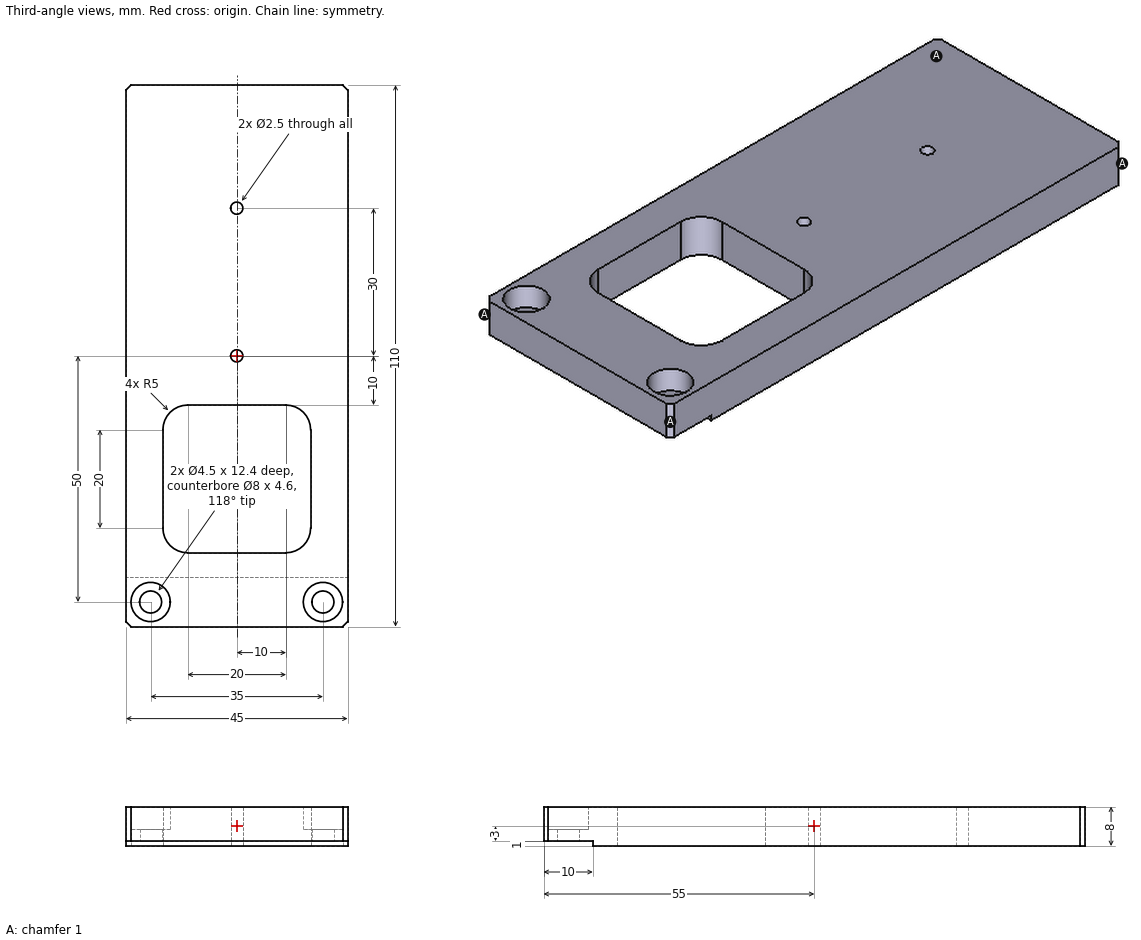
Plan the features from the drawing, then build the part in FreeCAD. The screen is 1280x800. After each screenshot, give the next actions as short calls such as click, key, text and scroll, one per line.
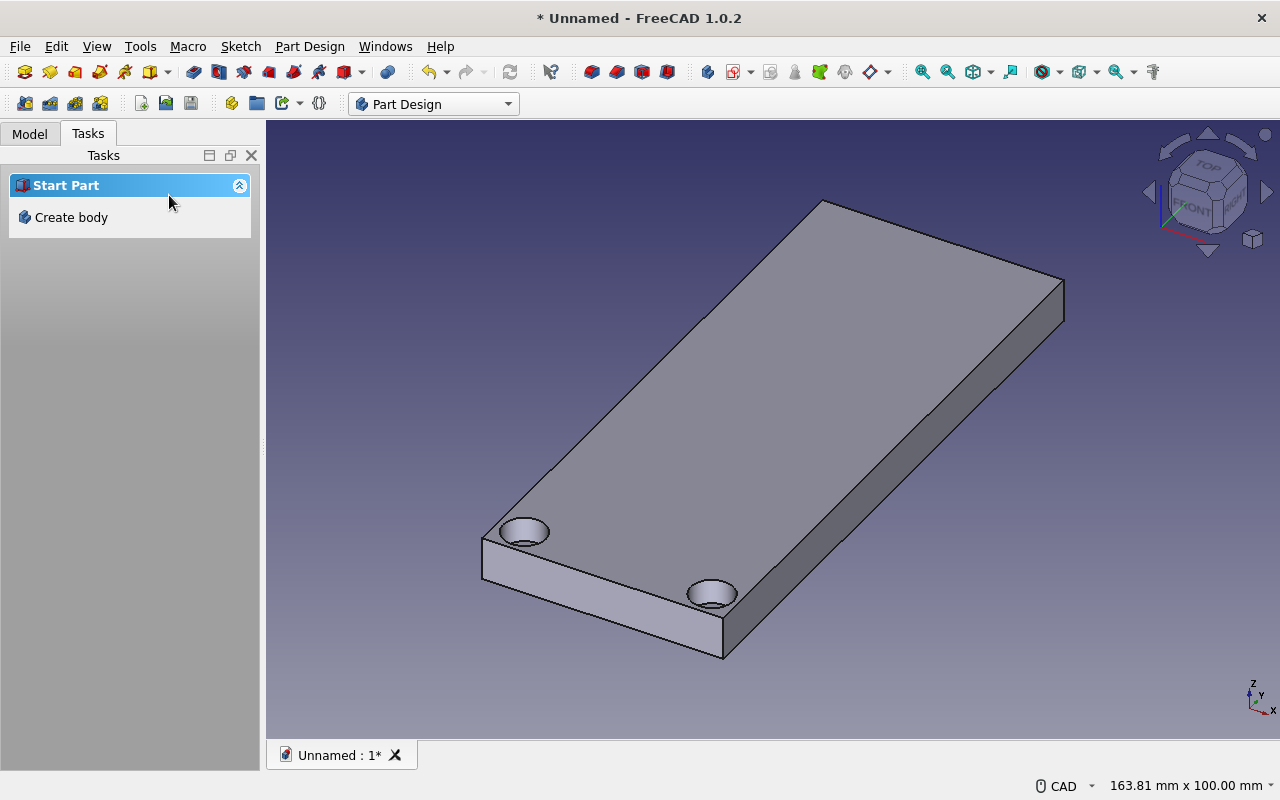
click(1040, 323)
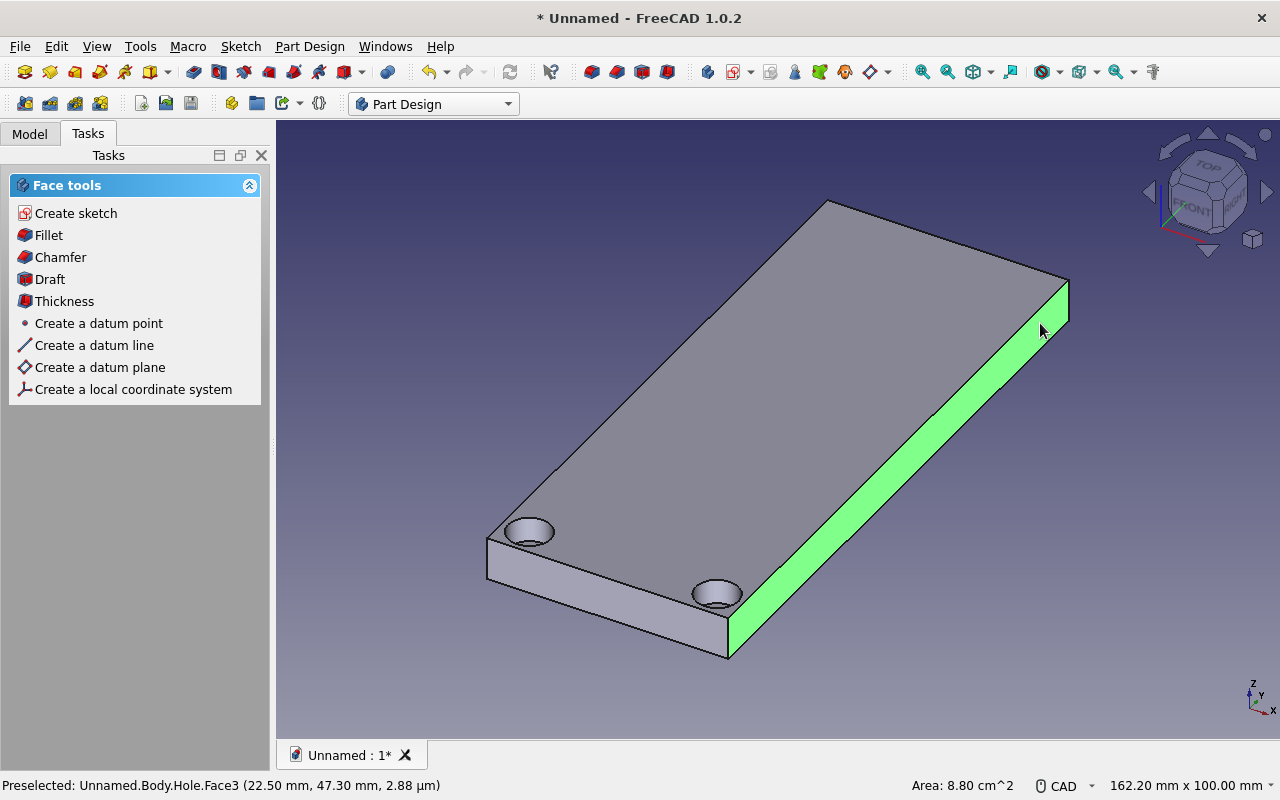
click(732, 72)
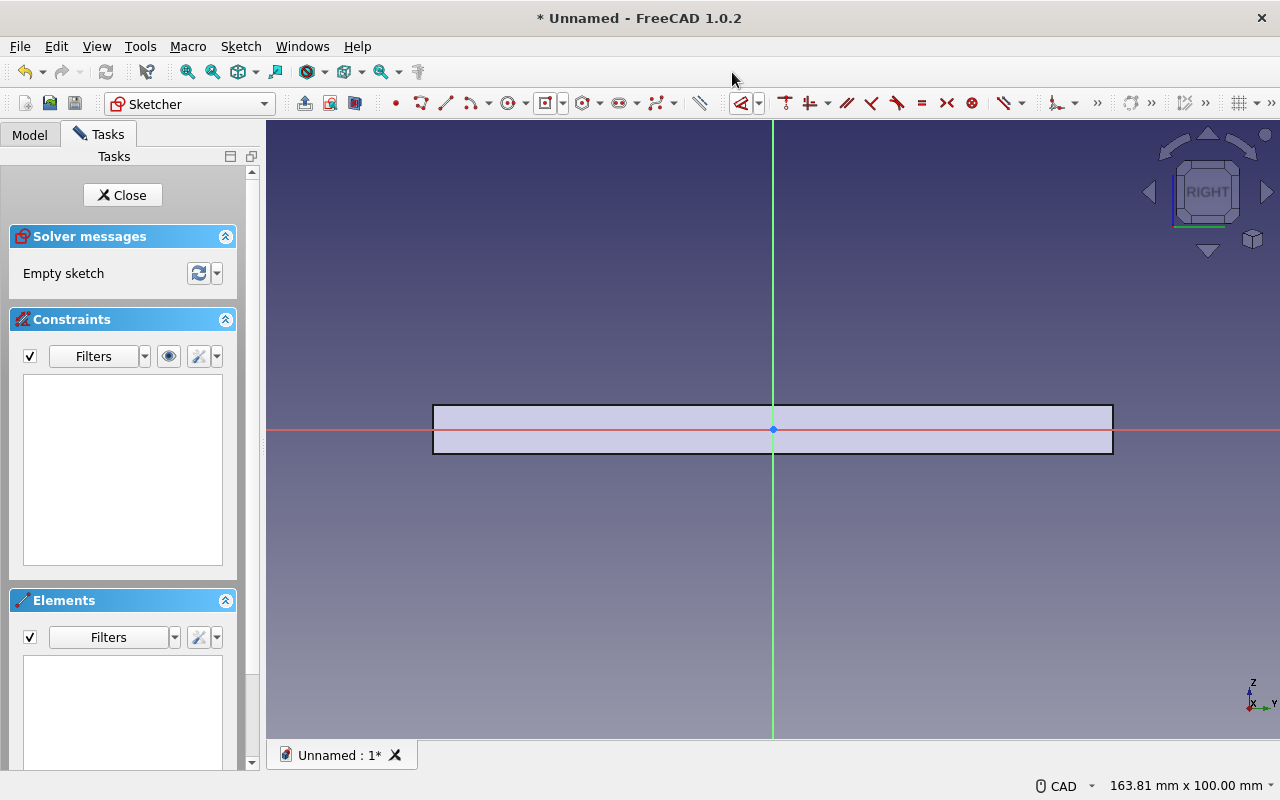
scroll(433, 454, up, 11)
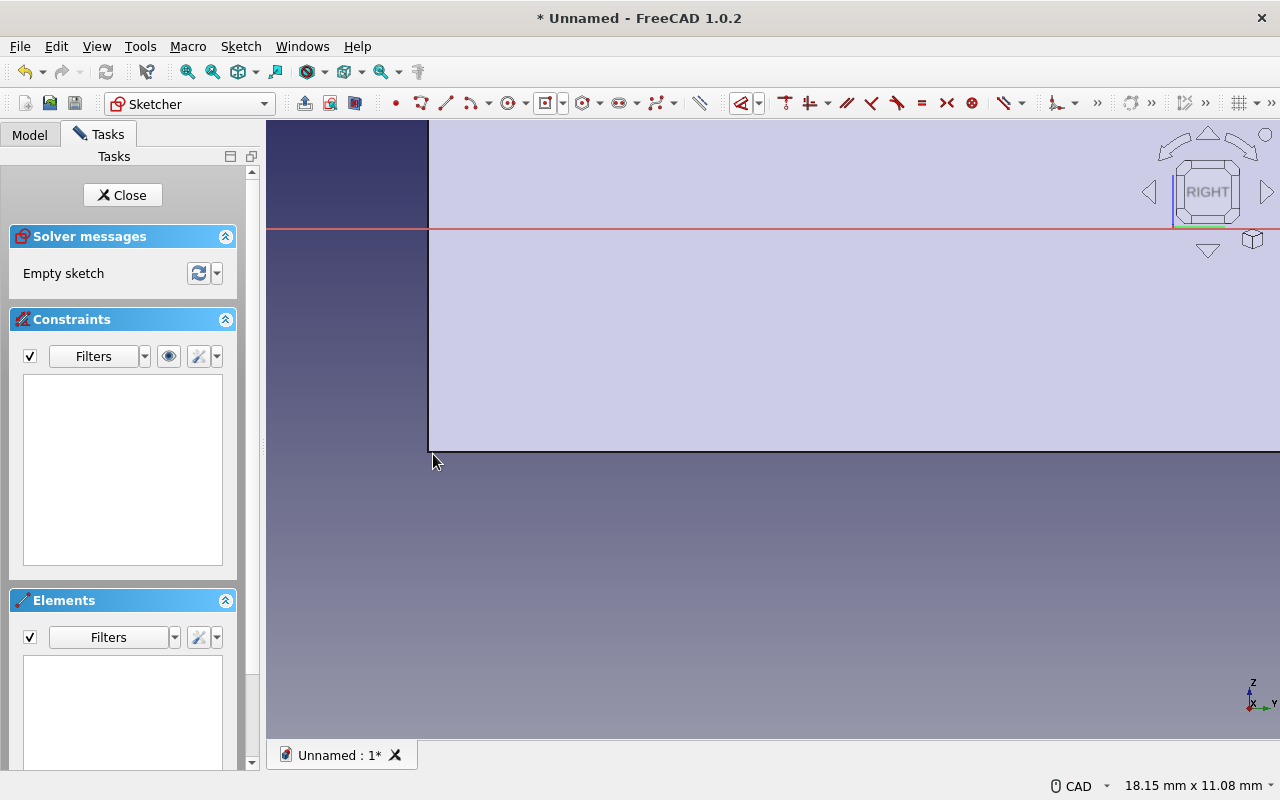
click(562, 104)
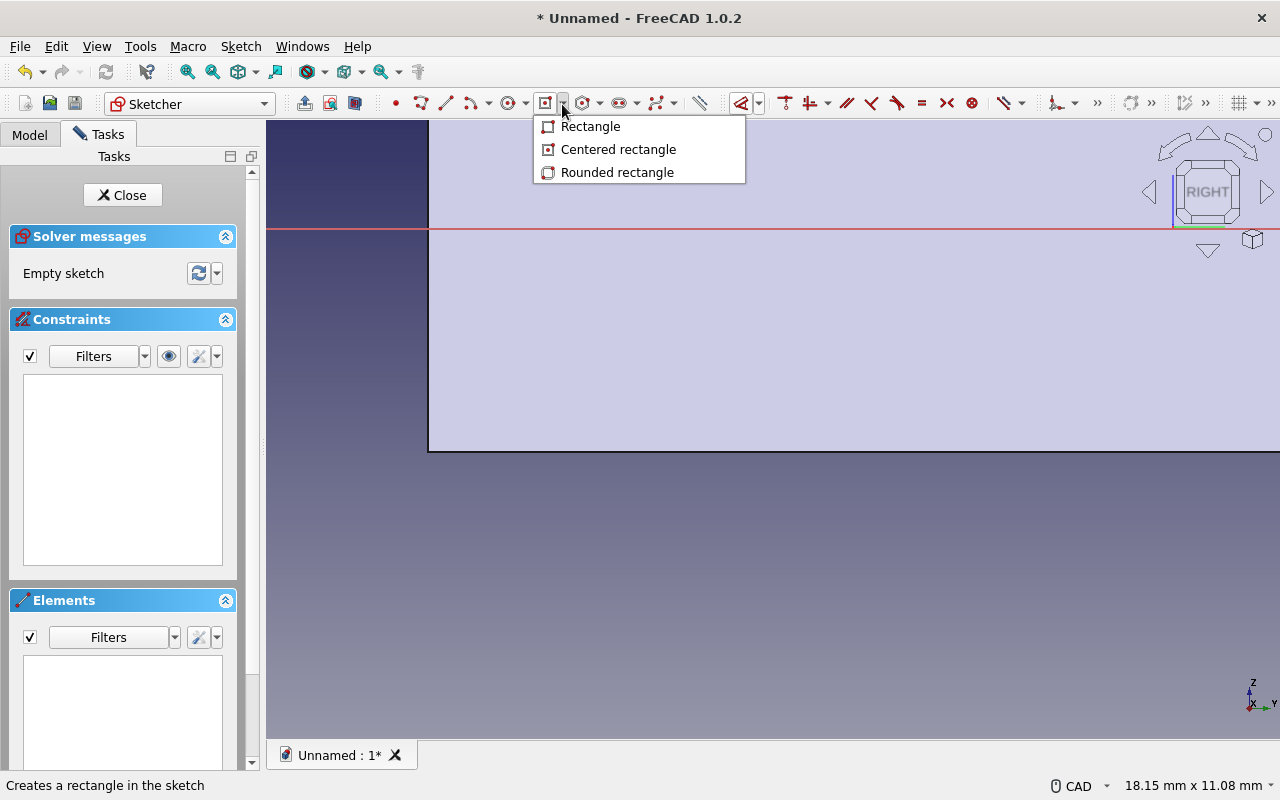
click(640, 126)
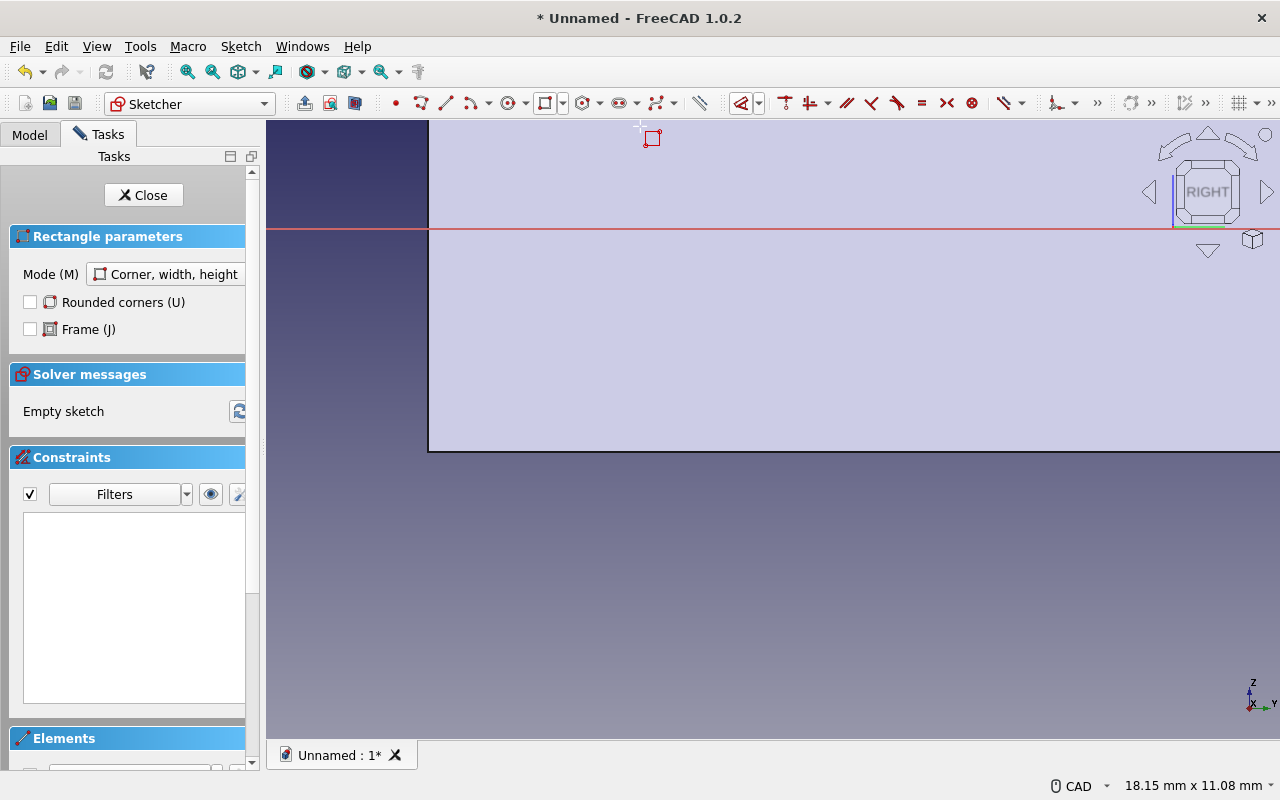
click(428, 396)
move(986, 452)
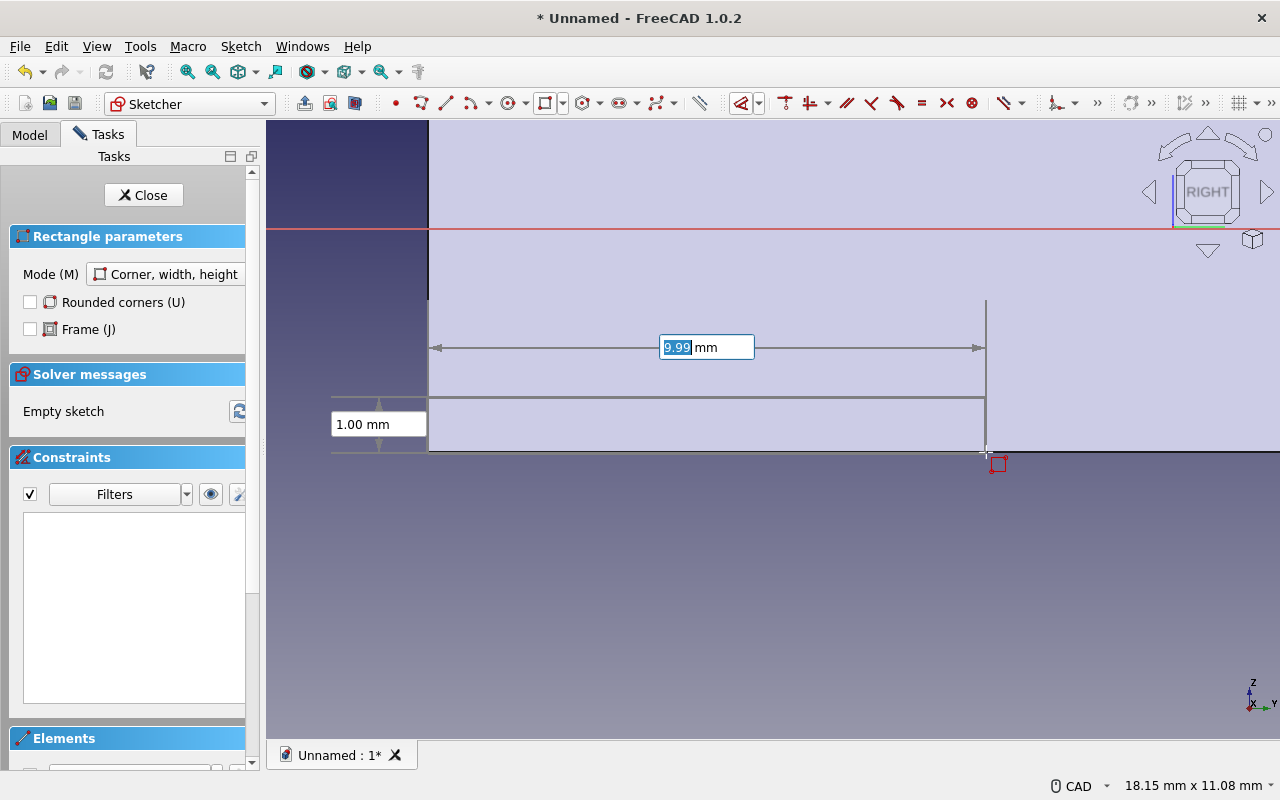
text(10)
key(Tab)
text(1)
key(Return)
key(Escape)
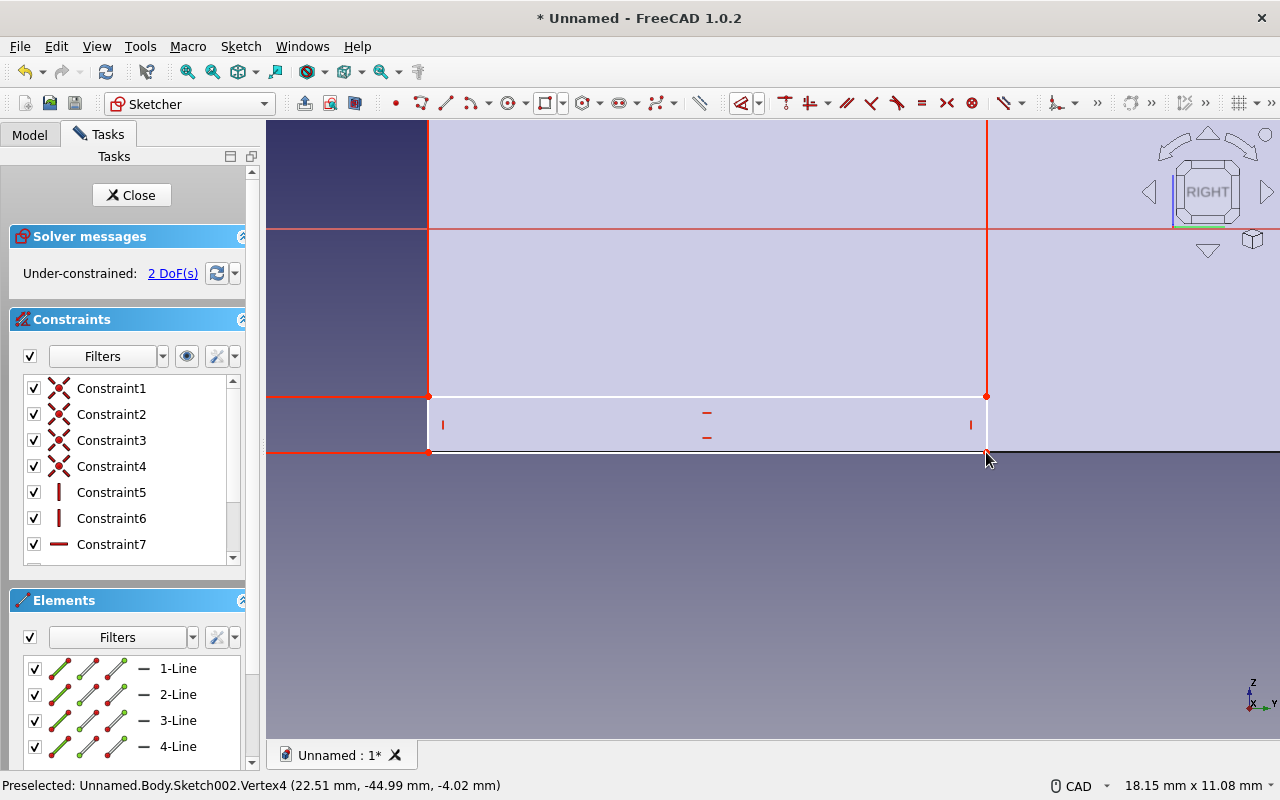
click(428, 397)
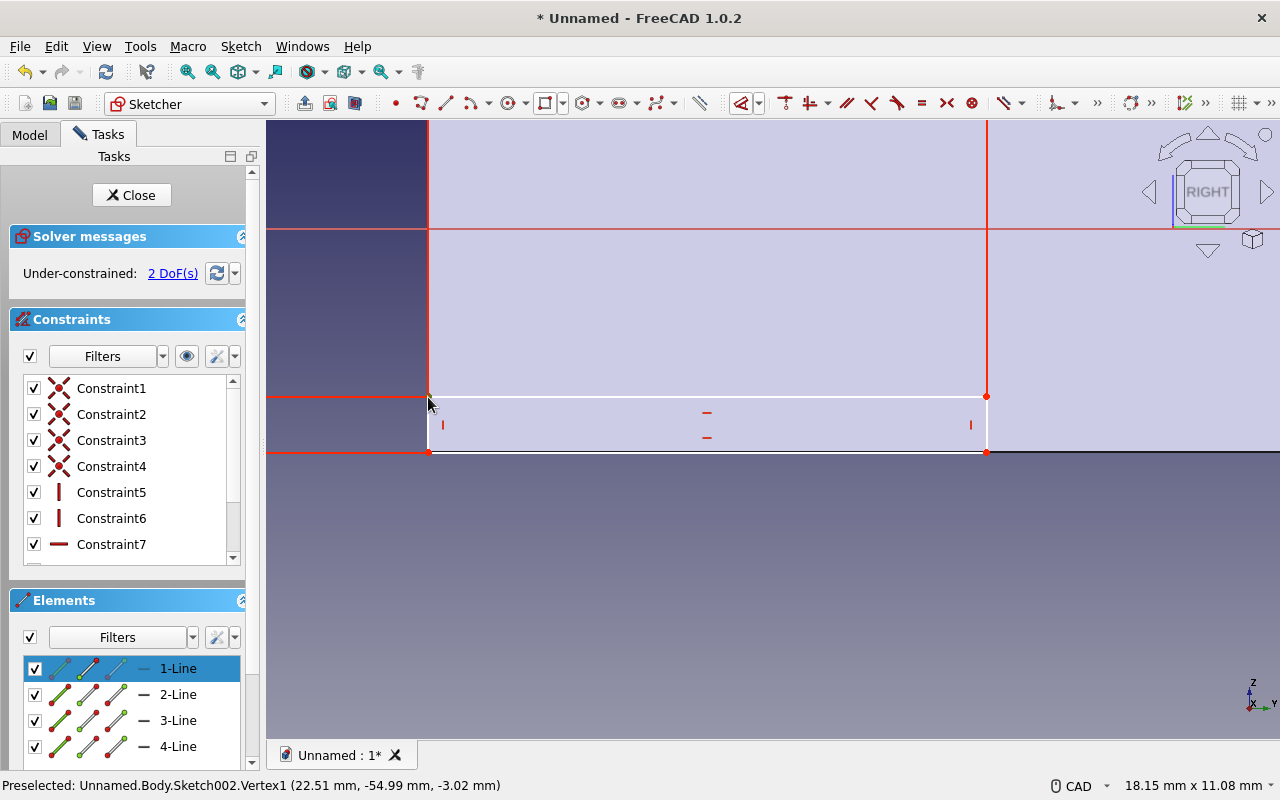
click(758, 104)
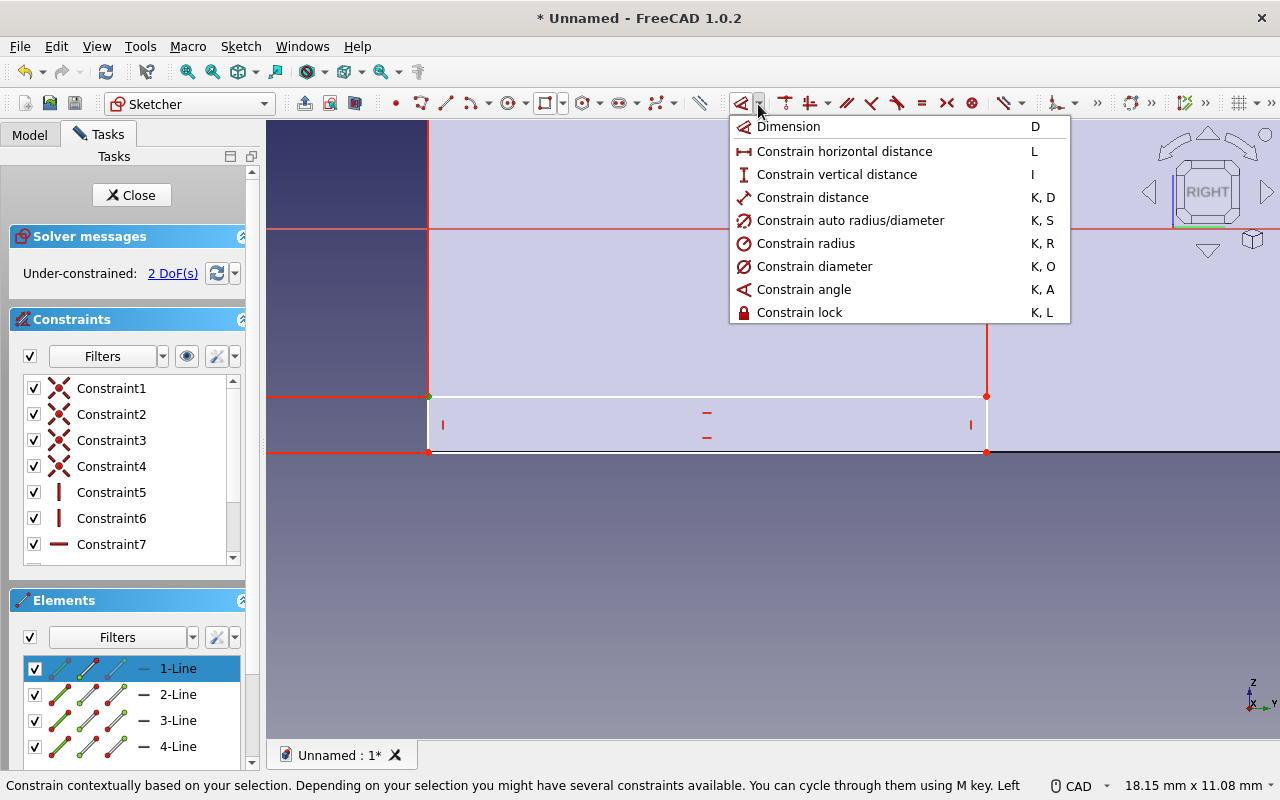
click(900, 174)